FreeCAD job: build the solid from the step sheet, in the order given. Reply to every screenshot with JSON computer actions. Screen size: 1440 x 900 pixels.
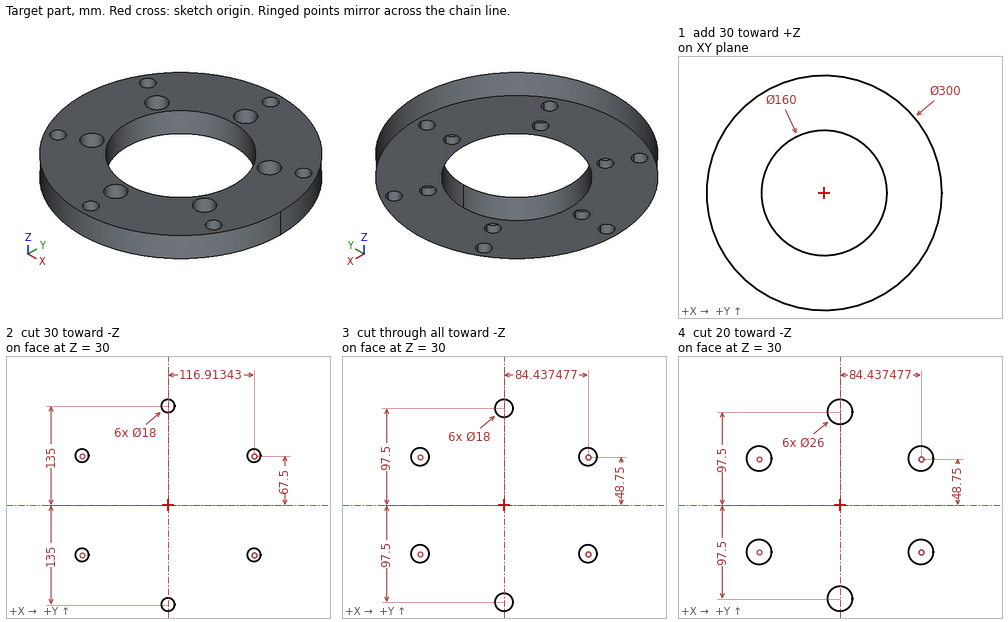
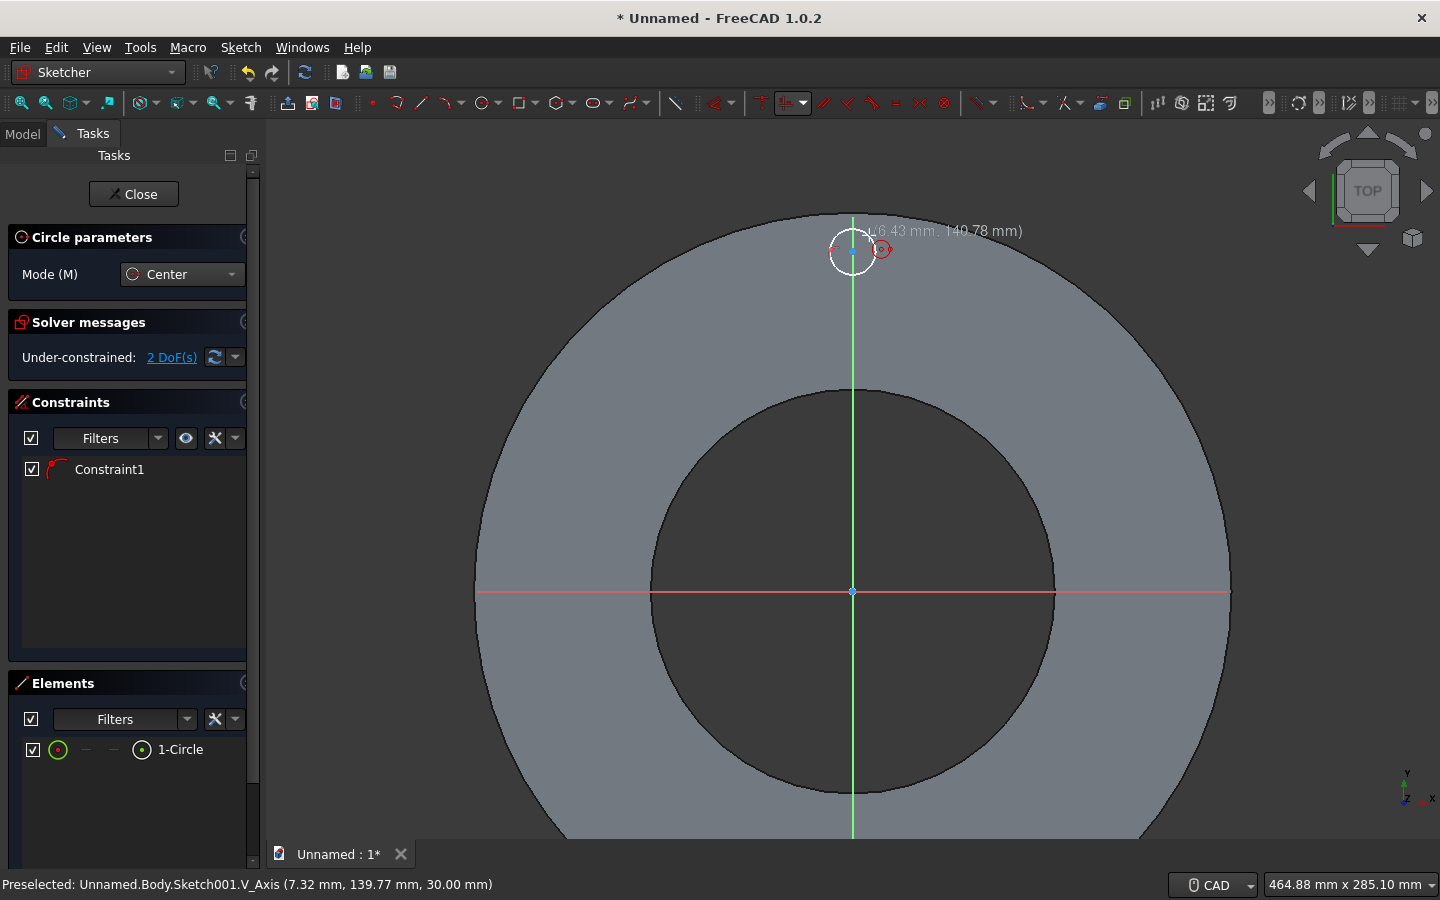
{"action": "left_click", "coordinate": [1148, 421]}
{"action": "left_click", "coordinate": [1164, 405]}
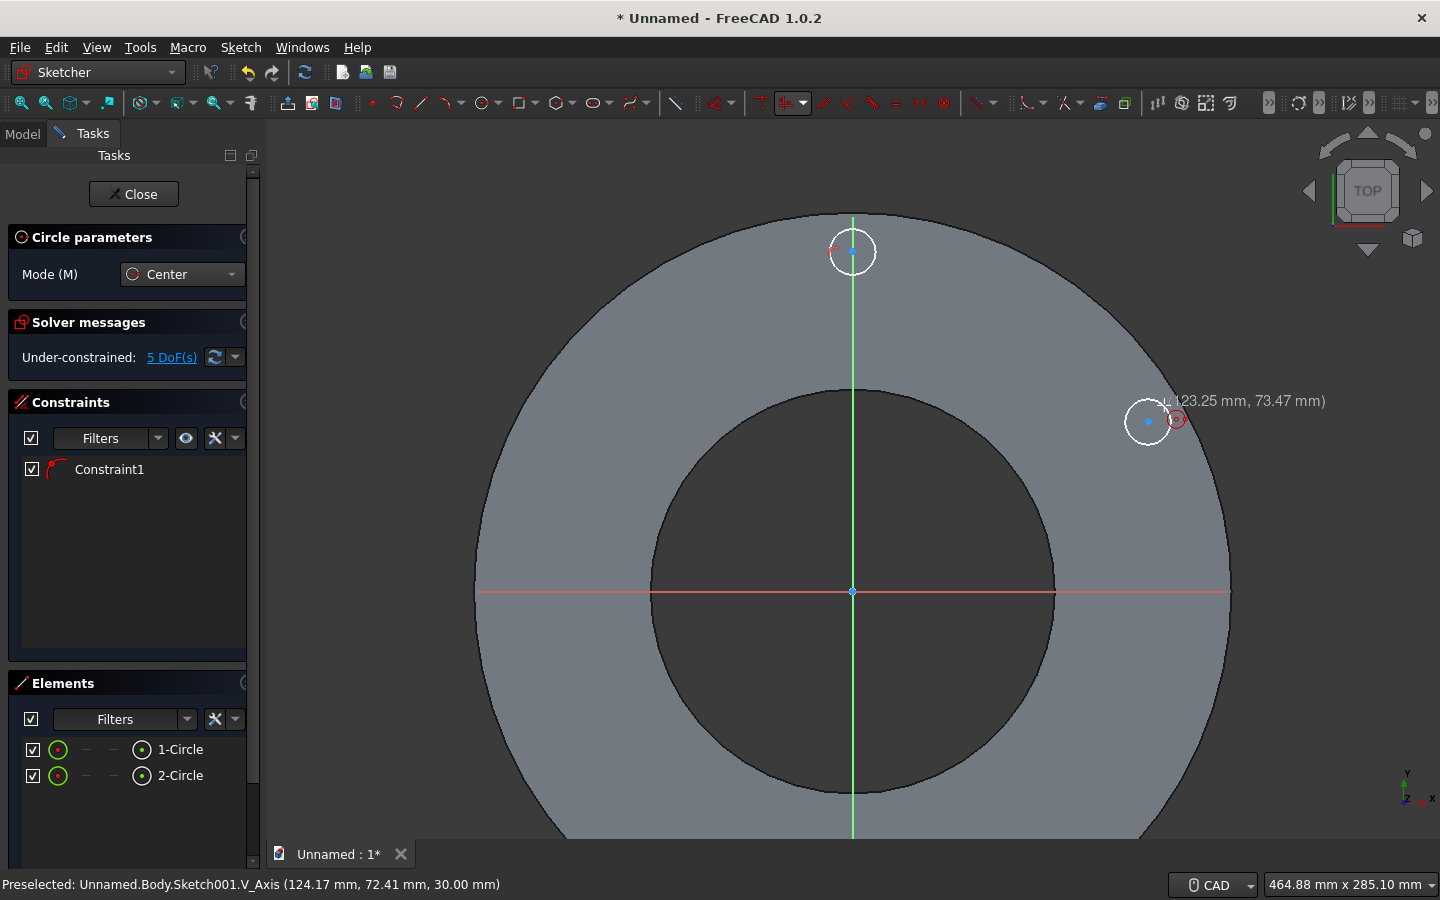
{"action": "left_click", "coordinate": [1148, 762]}
{"action": "left_click", "coordinate": [1164, 746]}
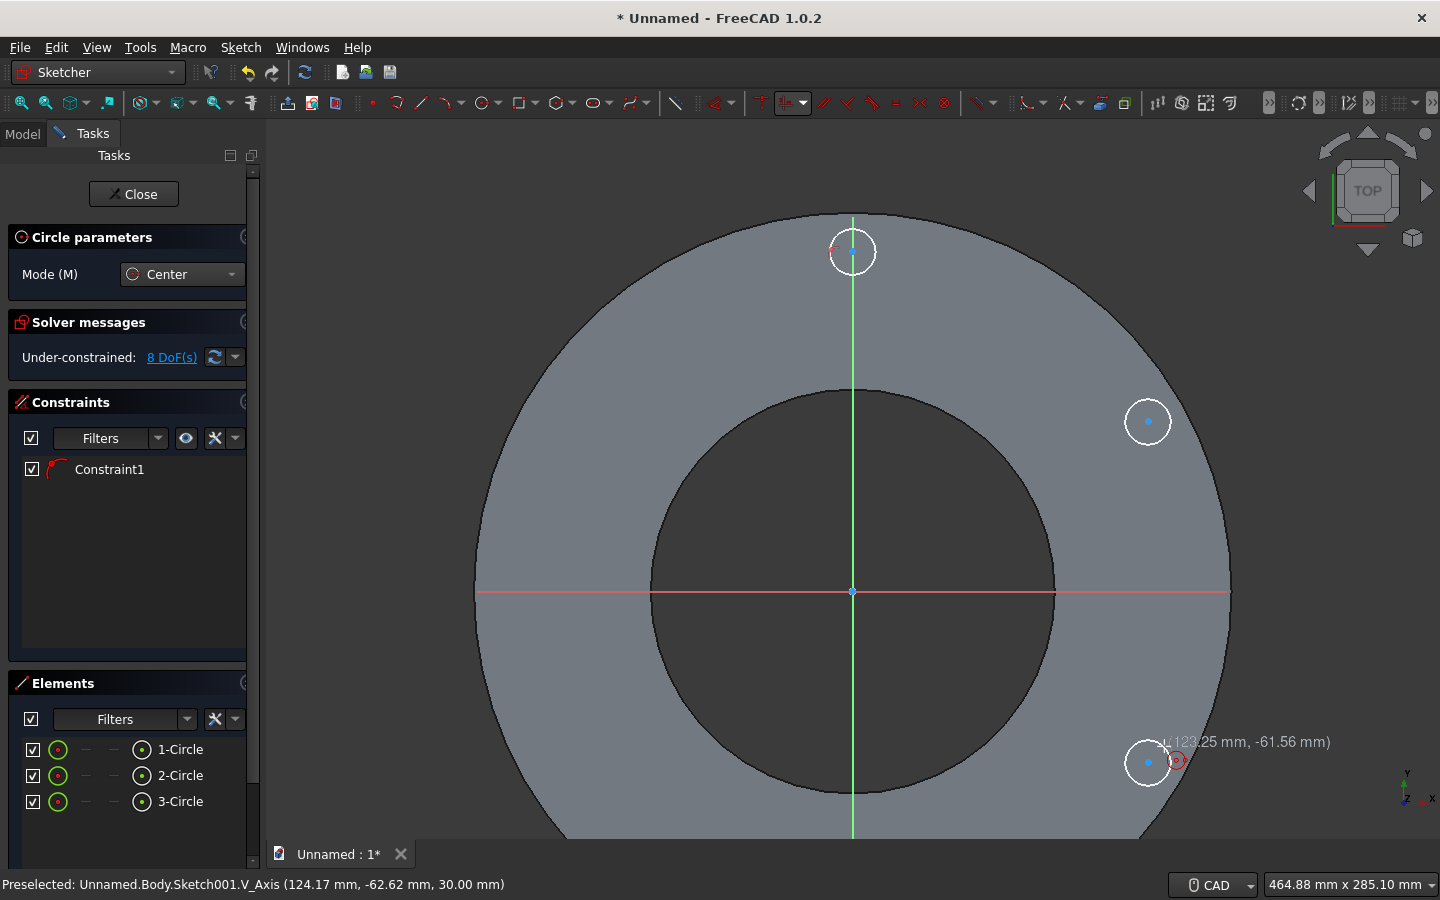
{"action": "scroll", "coordinate": [646, 250], "scroll_direction": "down", "scroll_amount": 2}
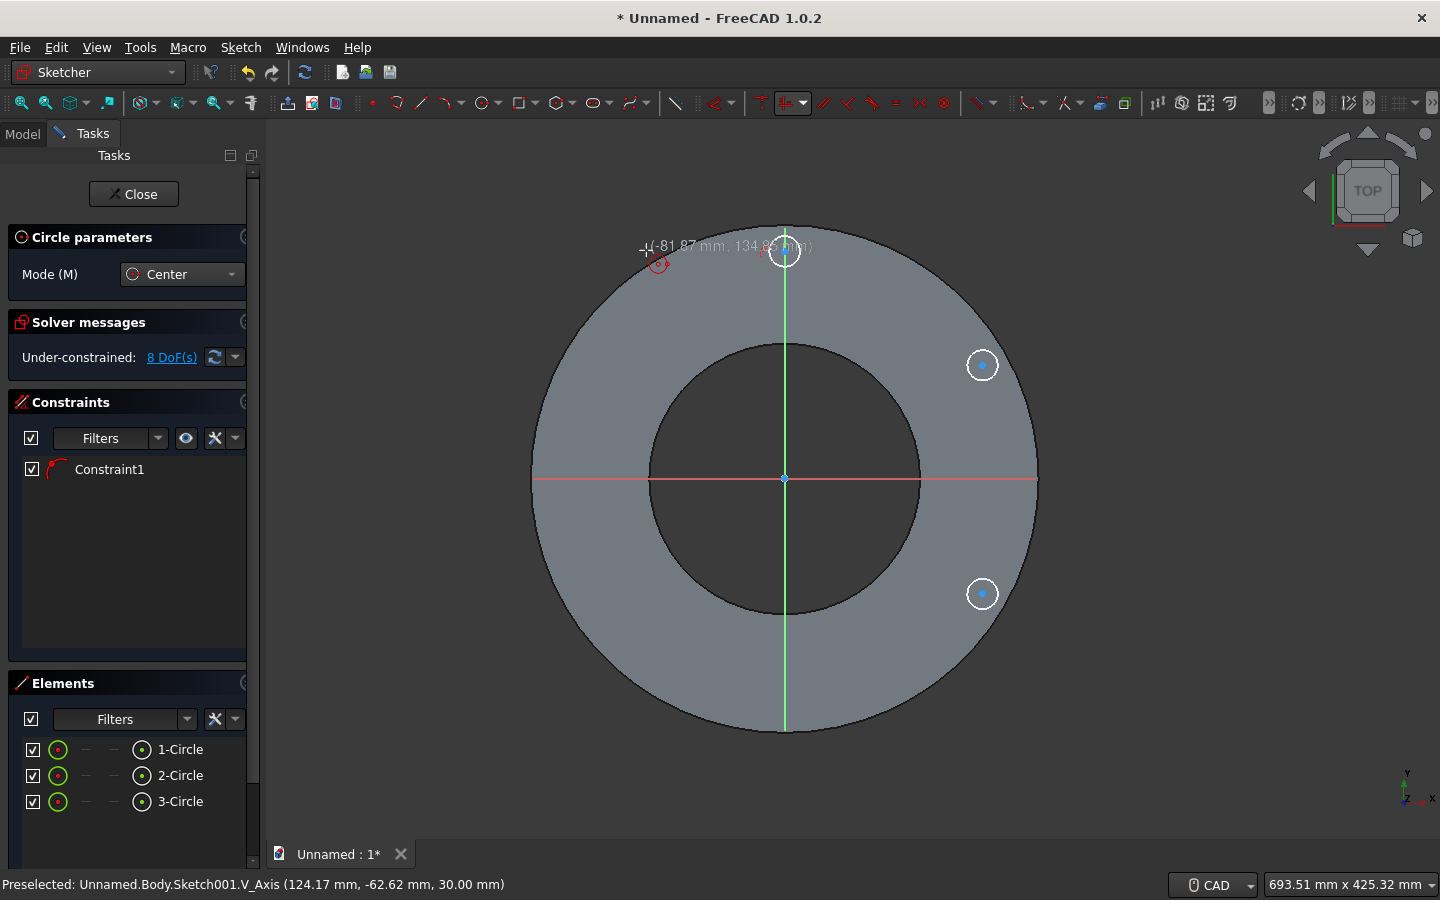
{"action": "scroll", "coordinate": [785, 708], "scroll_direction": "up", "scroll_amount": 2}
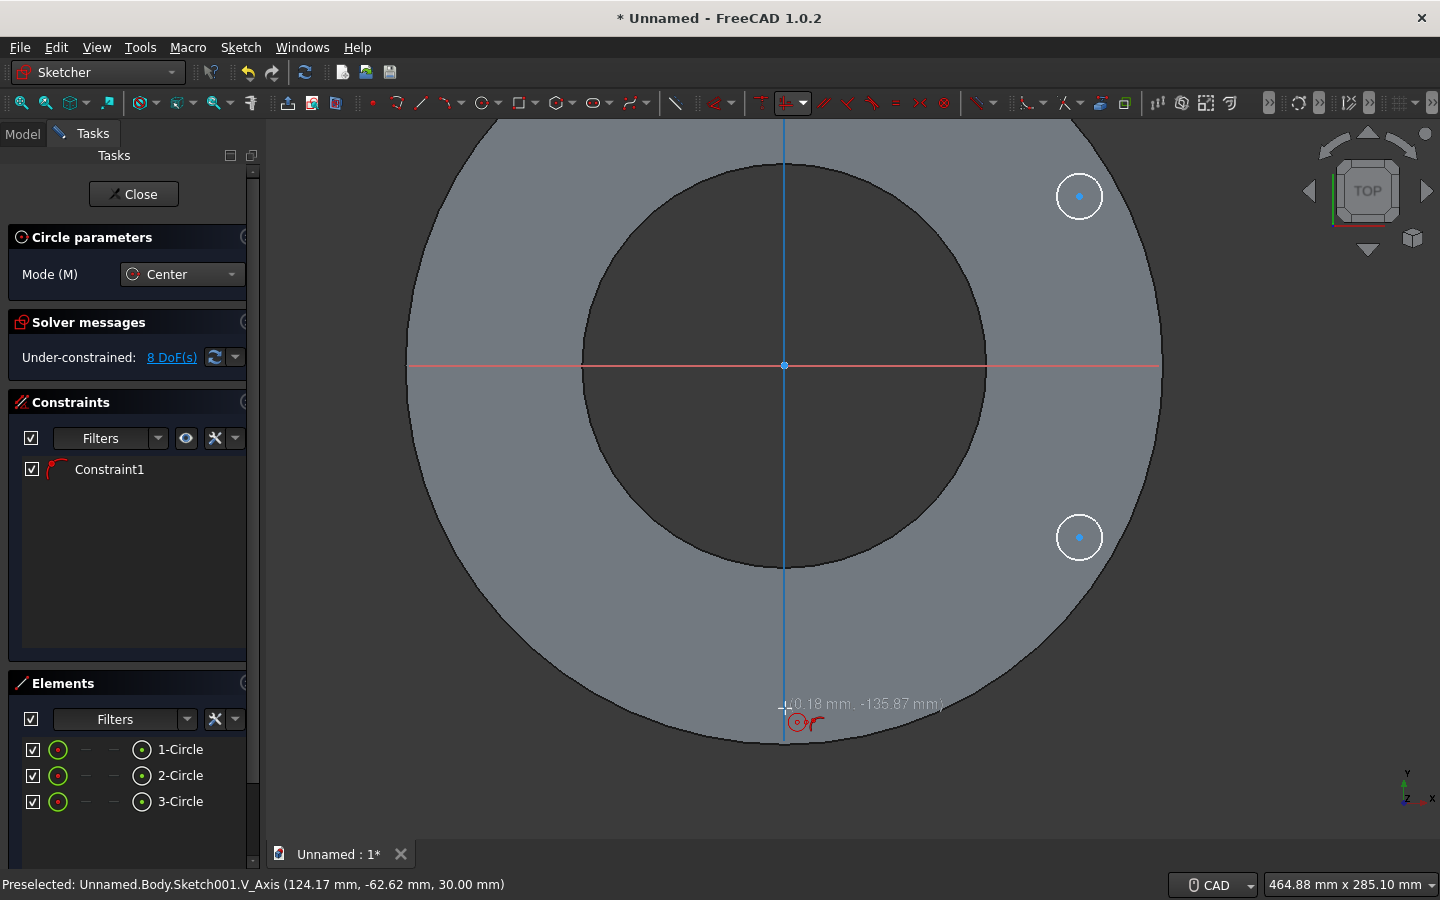
{"action": "left_click", "coordinate": [784, 707]}
{"action": "left_click", "coordinate": [800, 691]}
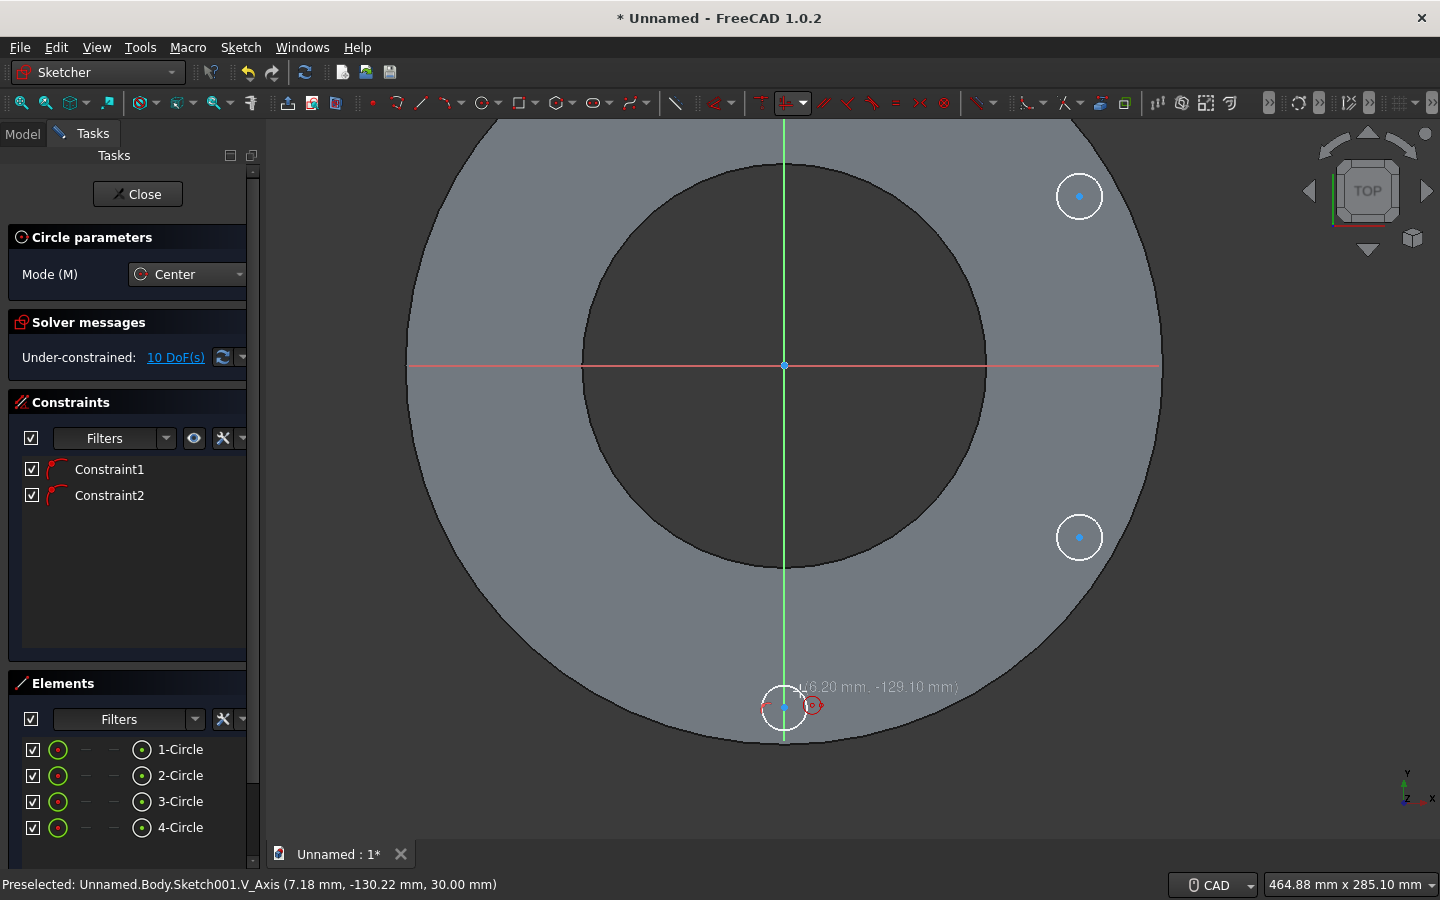
{"action": "left_click", "coordinate": [489, 536]}
{"action": "left_click", "coordinate": [505, 520]}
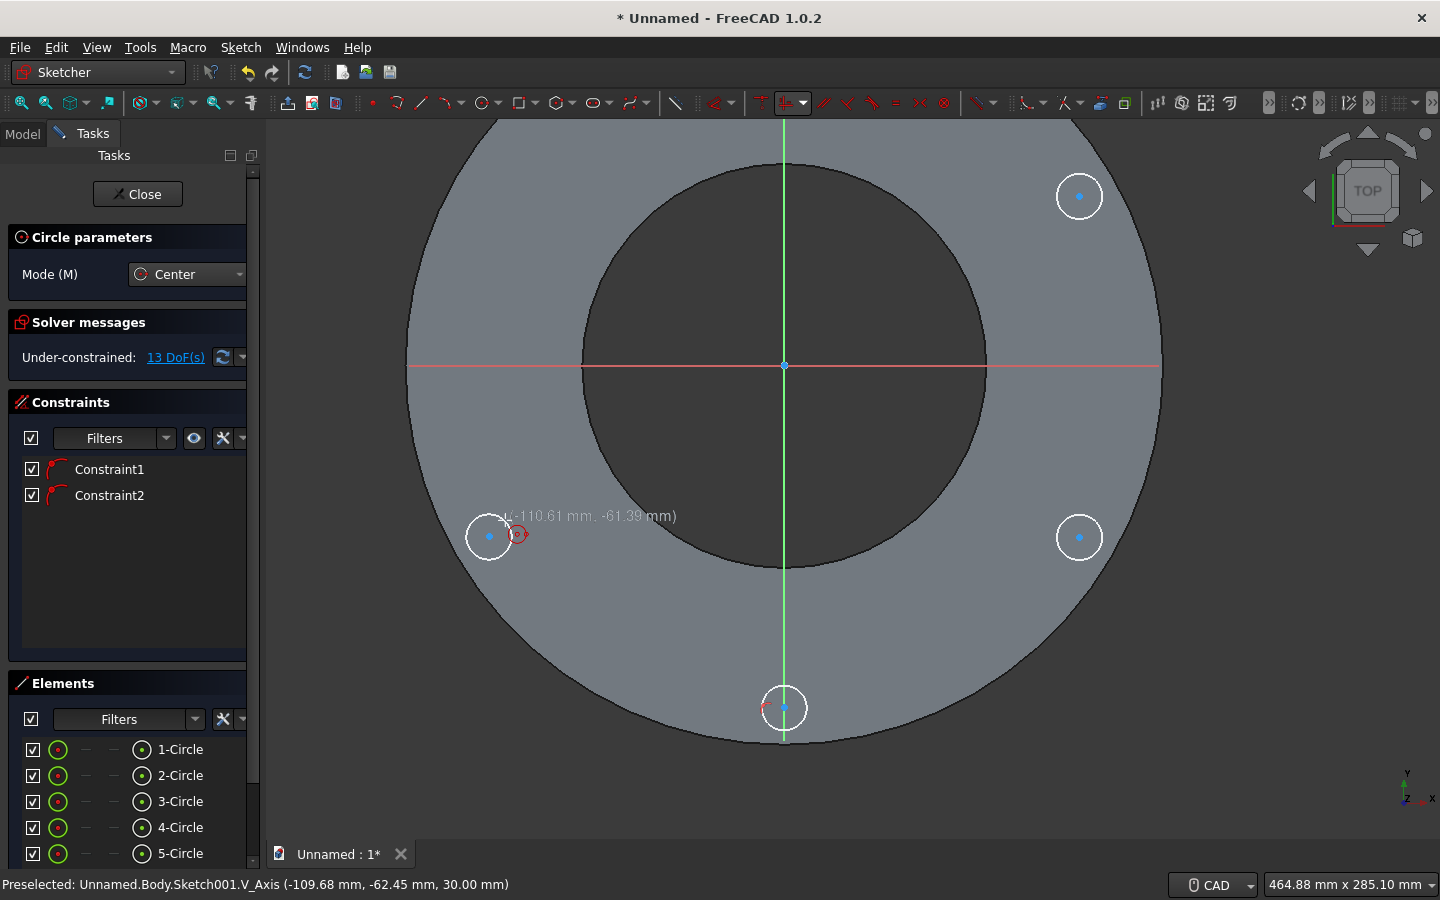
{"action": "left_click", "coordinate": [489, 196]}
{"action": "left_click", "coordinate": [505, 179]}
{"action": "key", "text": "Escape"}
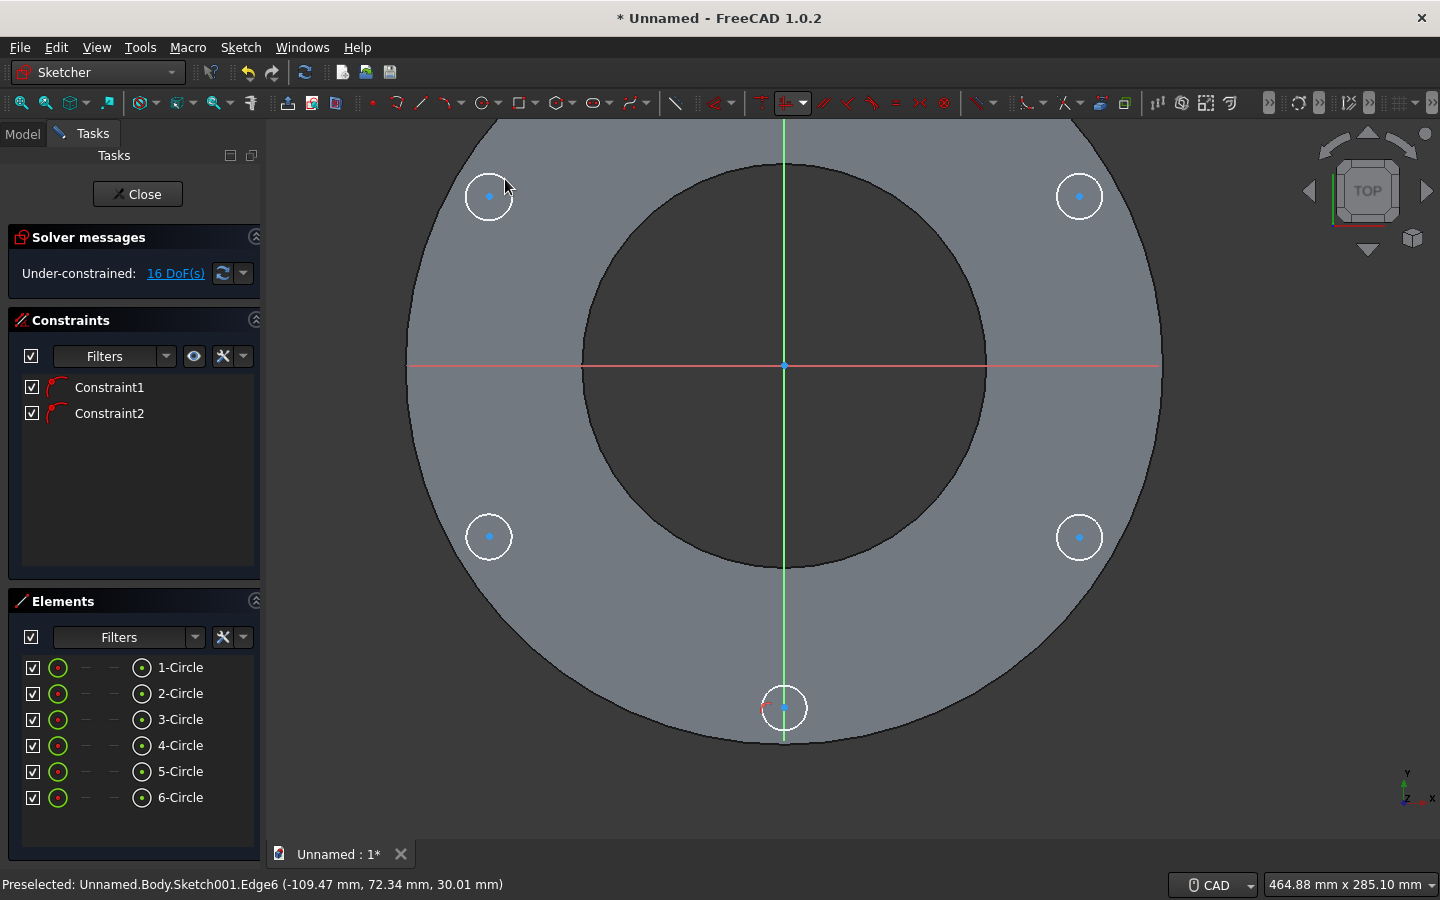
{"action": "scroll", "coordinate": [785, 709], "scroll_direction": "down", "scroll_amount": 2}